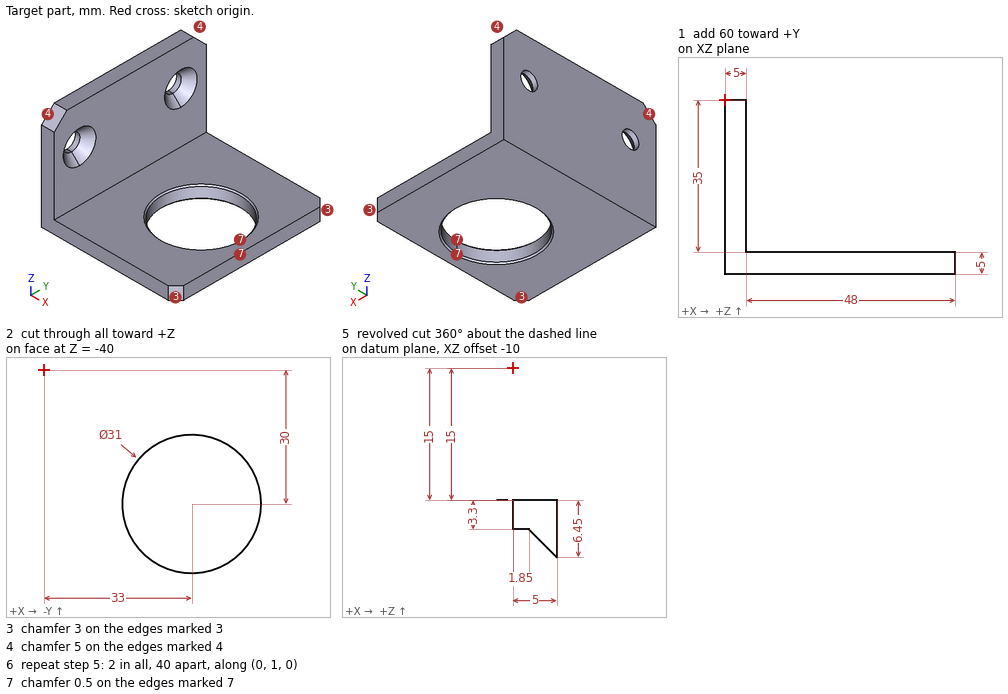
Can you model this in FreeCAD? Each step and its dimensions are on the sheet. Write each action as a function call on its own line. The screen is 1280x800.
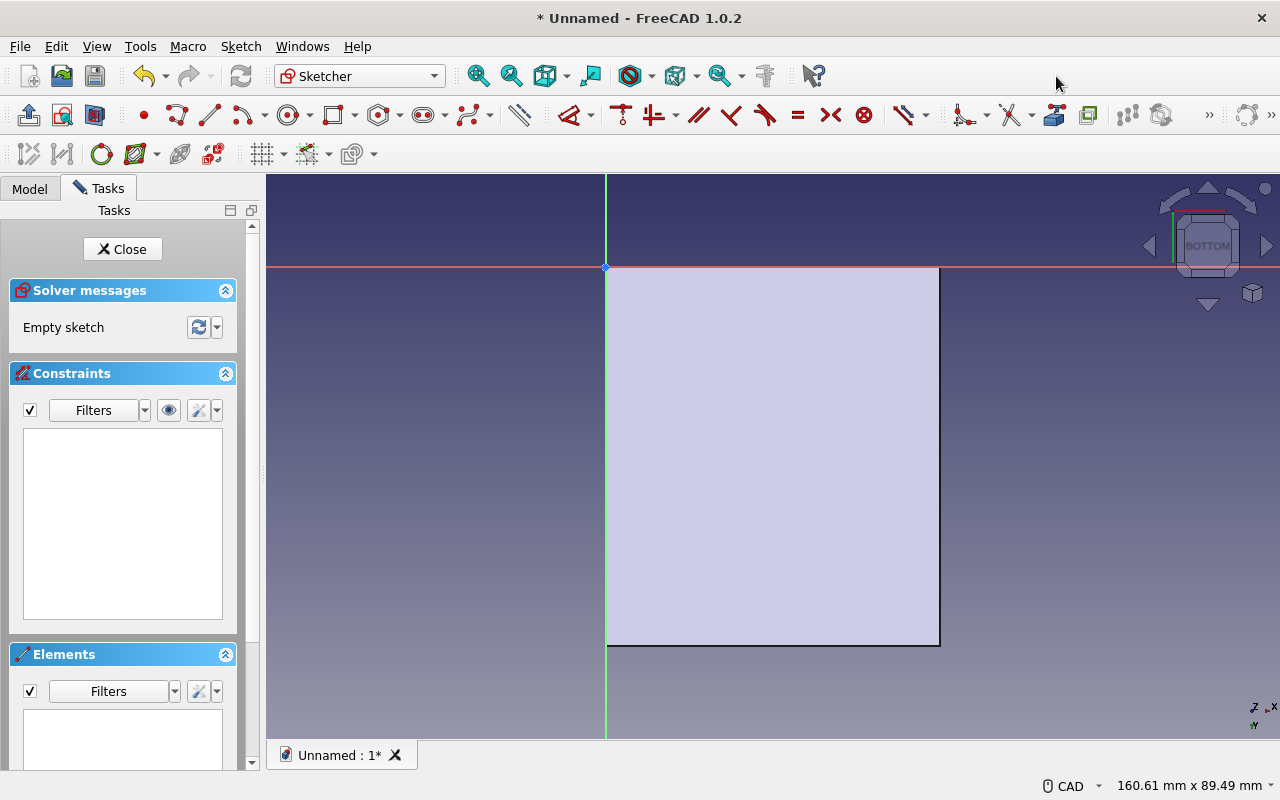
key(g)
key(c)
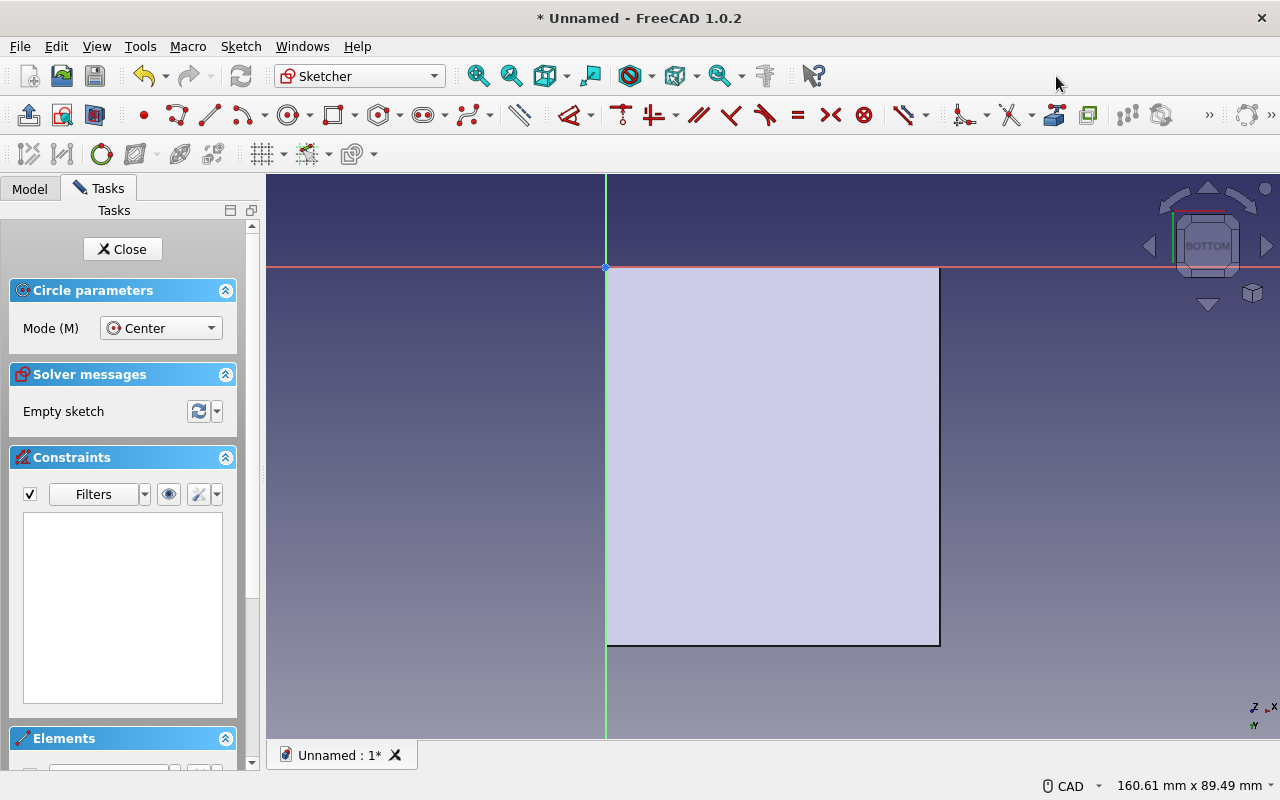
click(814, 456)
click(883, 387)
key(Escape)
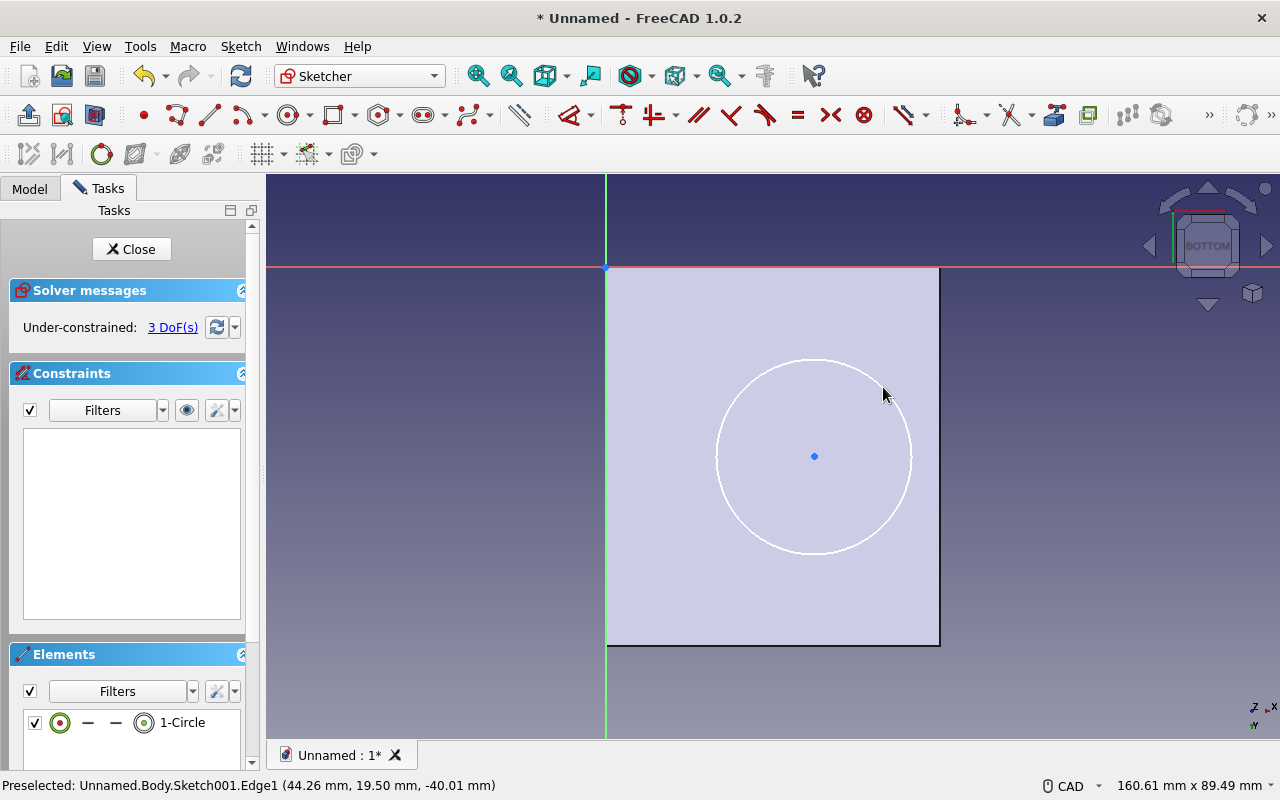
click(883, 388)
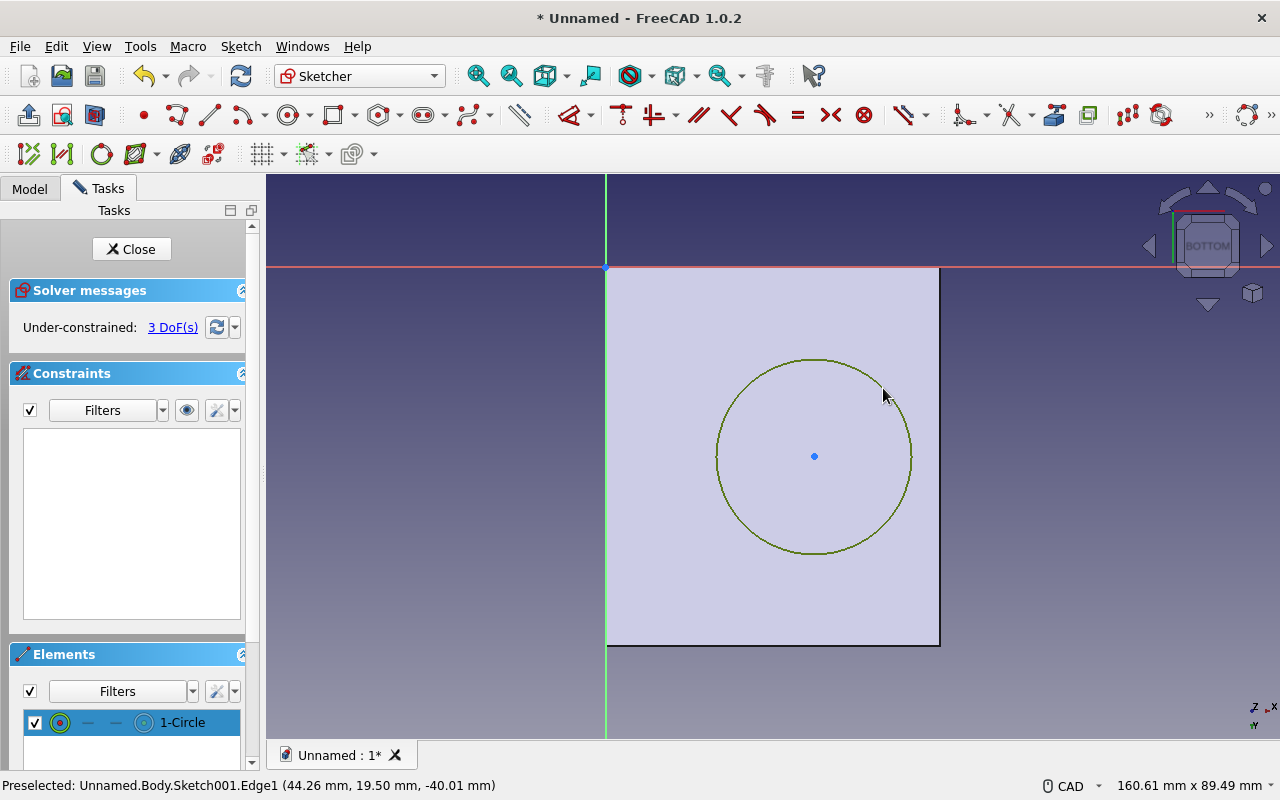
key(k)
key(o)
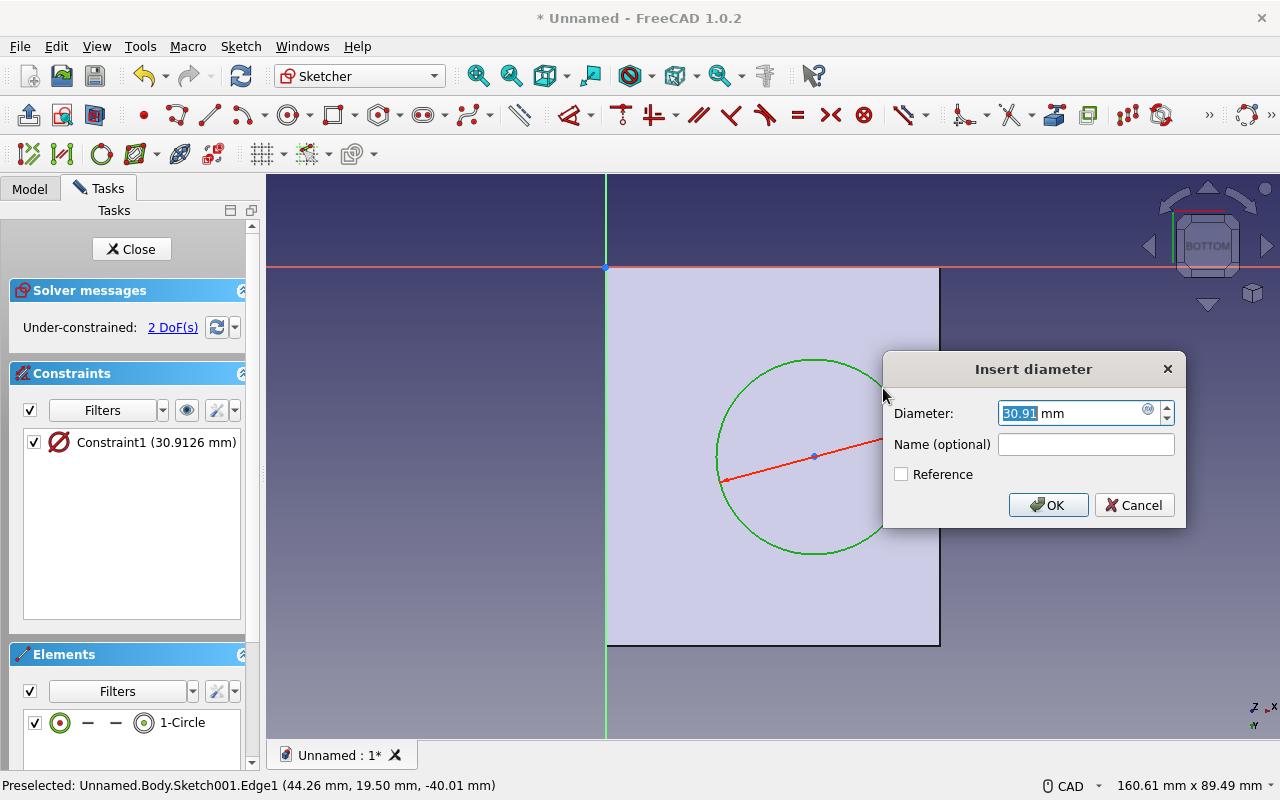
text(31)
key(Return)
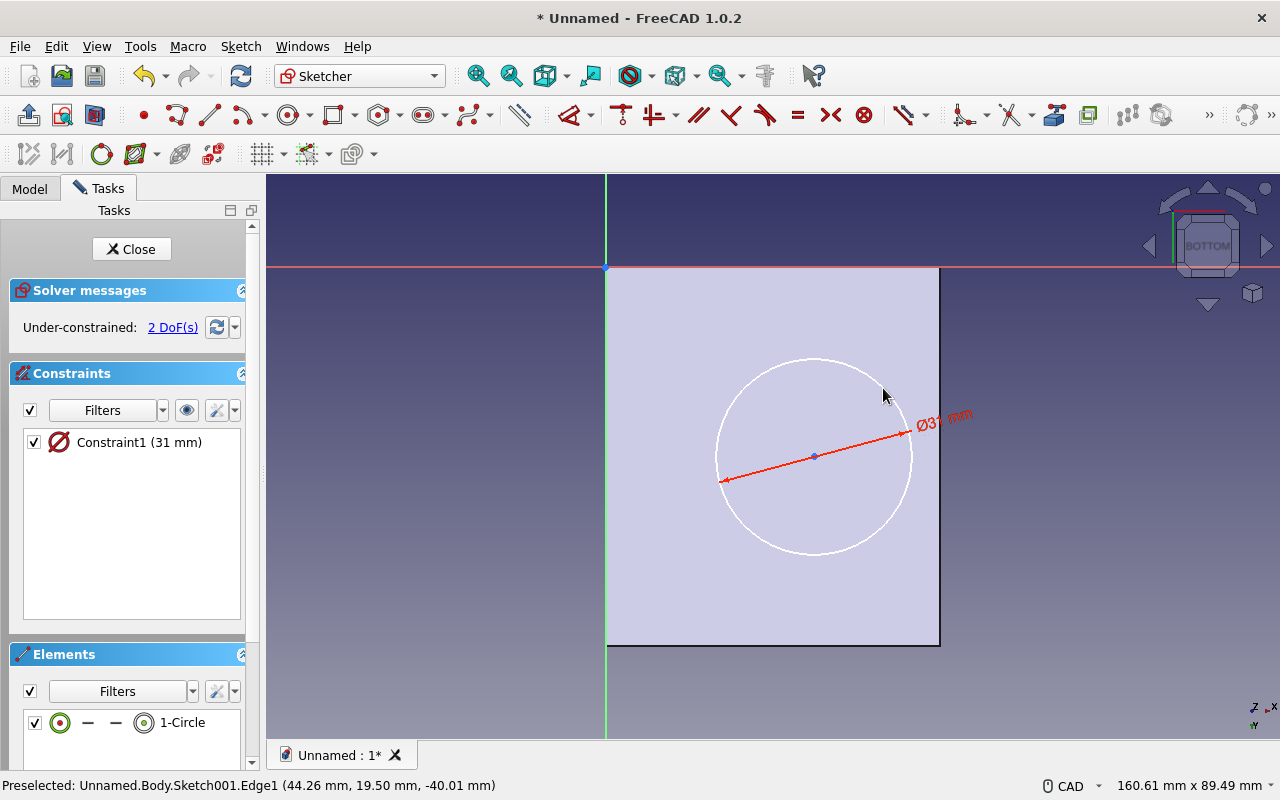
click(814, 457)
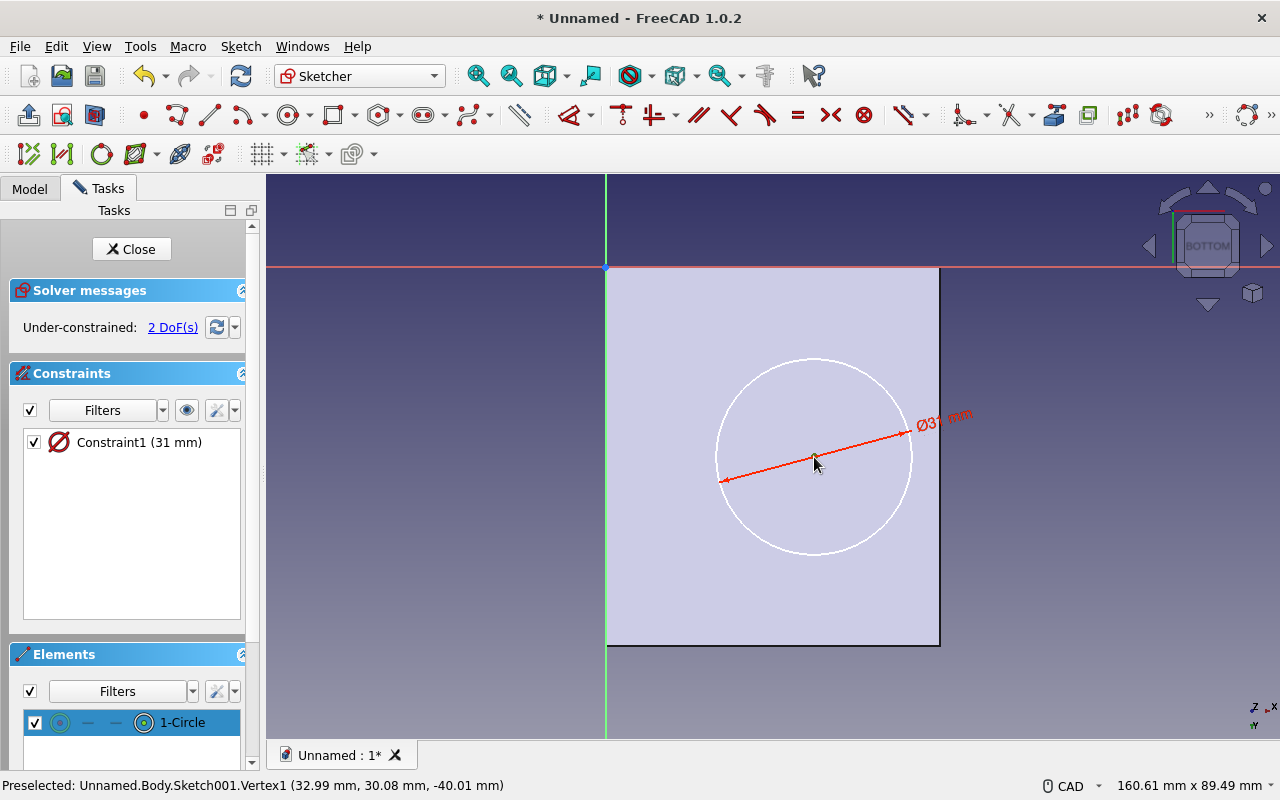
key(l)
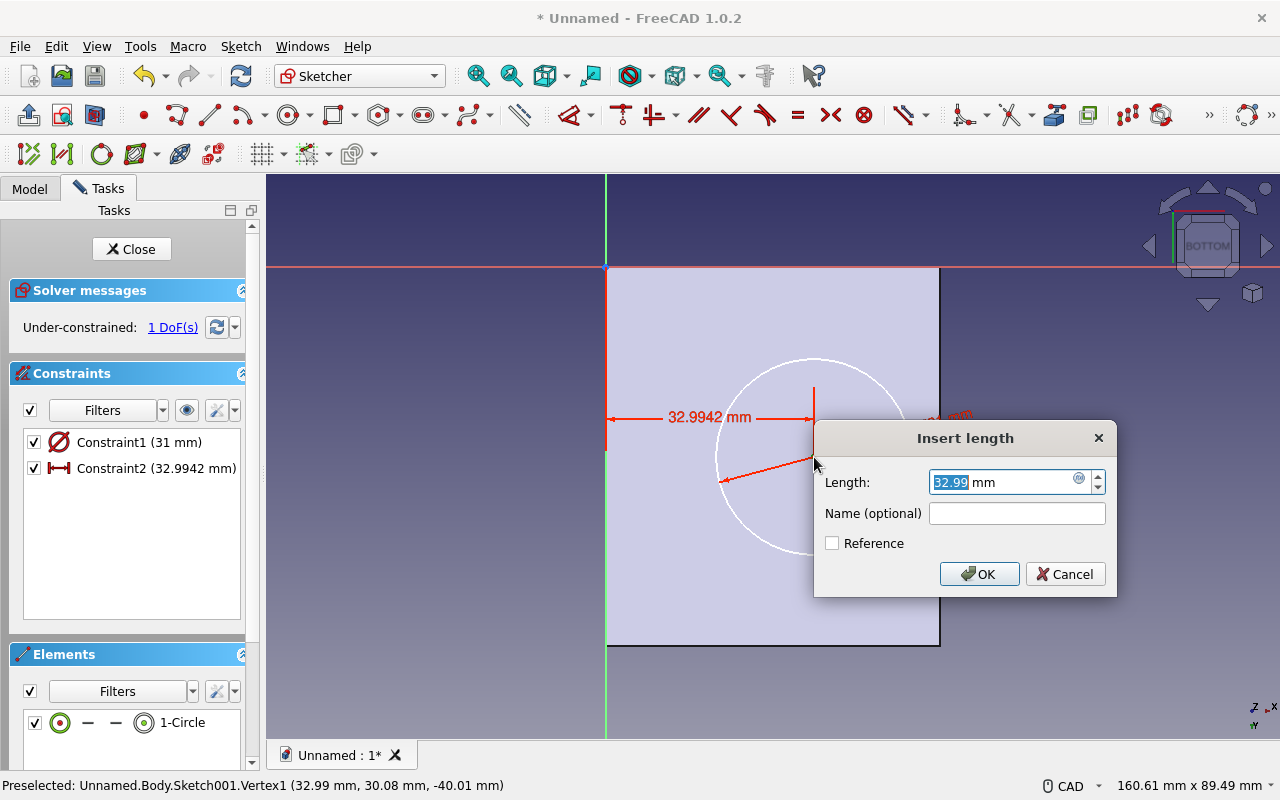
text(33)
key(Return)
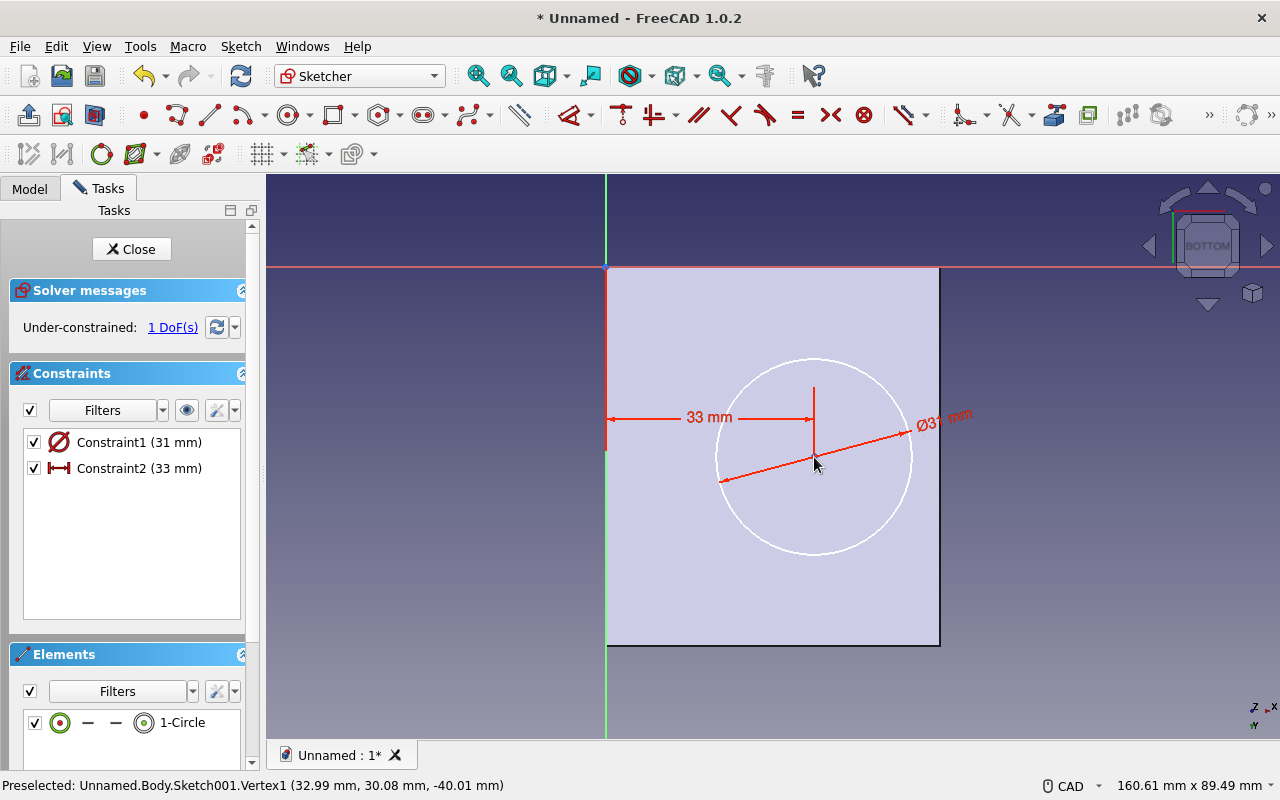
click(814, 457)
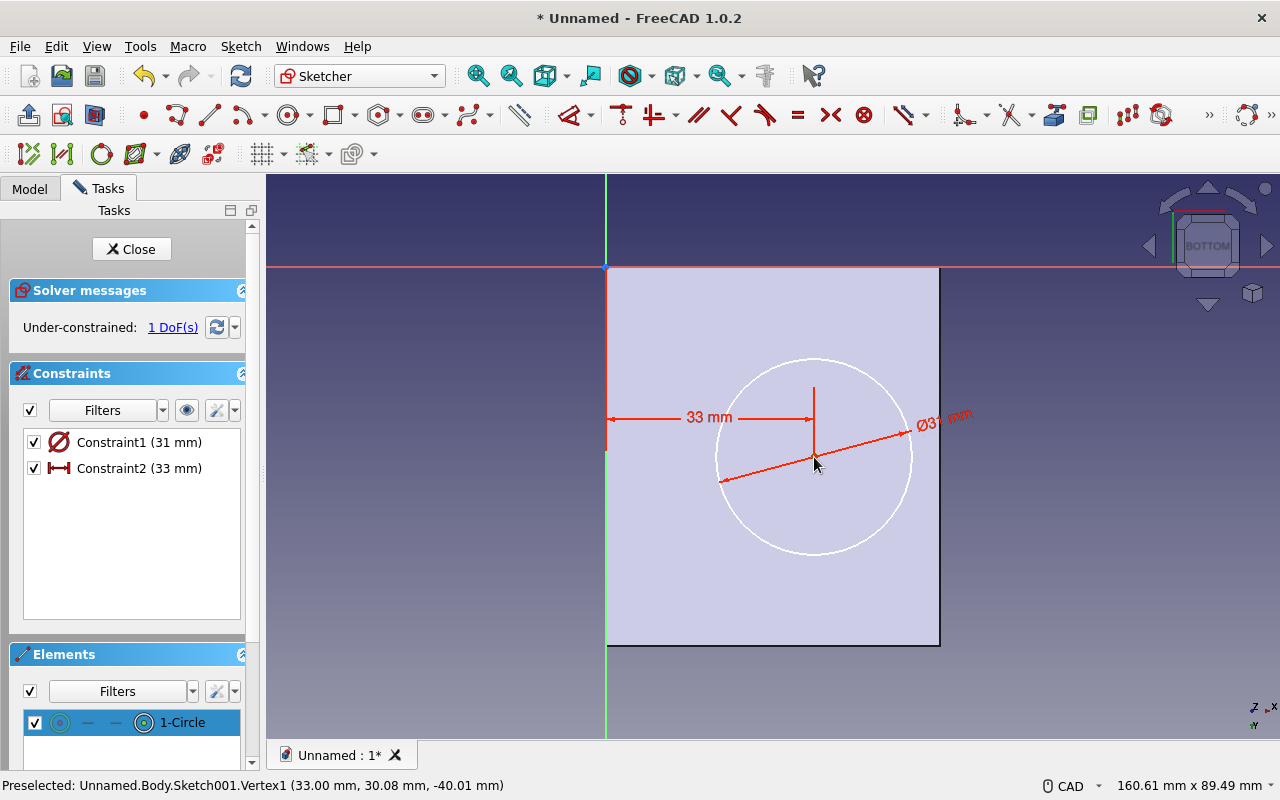
key(i)